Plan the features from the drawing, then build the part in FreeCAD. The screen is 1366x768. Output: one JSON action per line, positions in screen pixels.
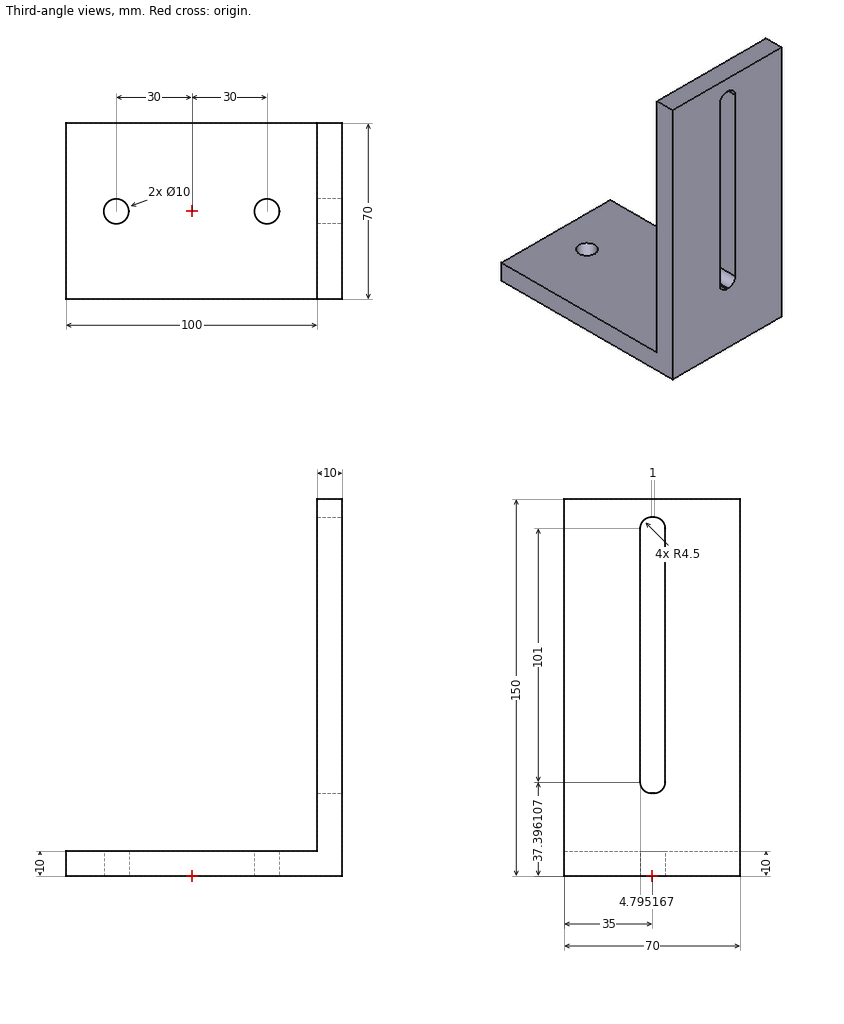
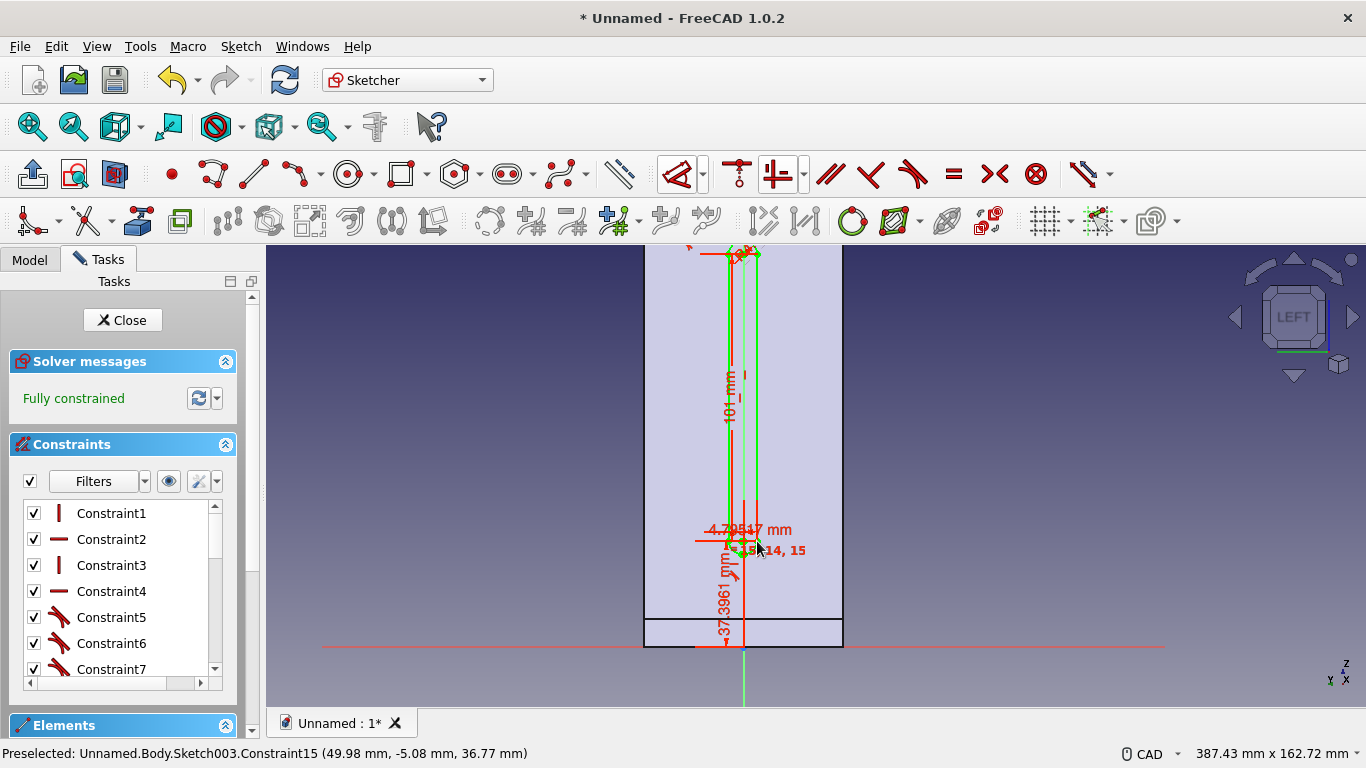
{"action": "left_click", "coordinate": [123, 320]}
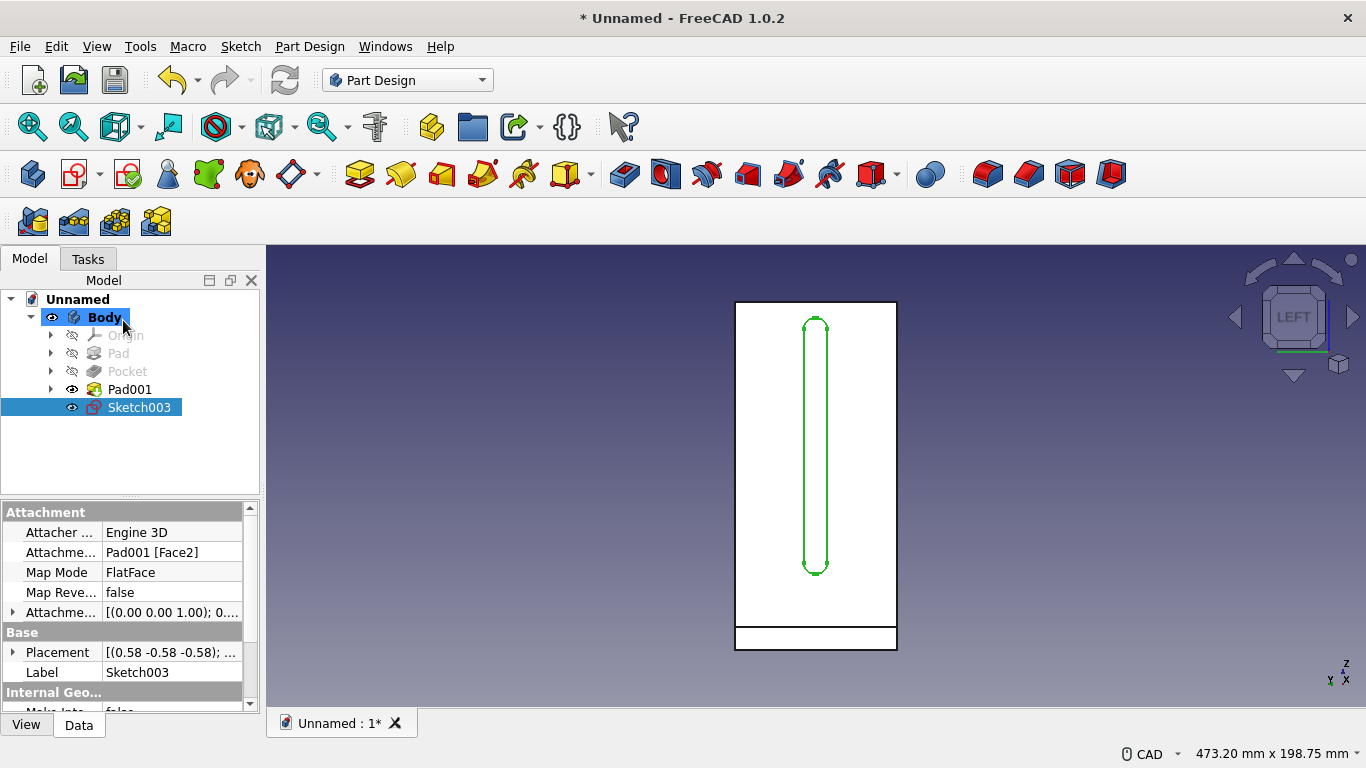
{"action": "left_click", "coordinate": [625, 174]}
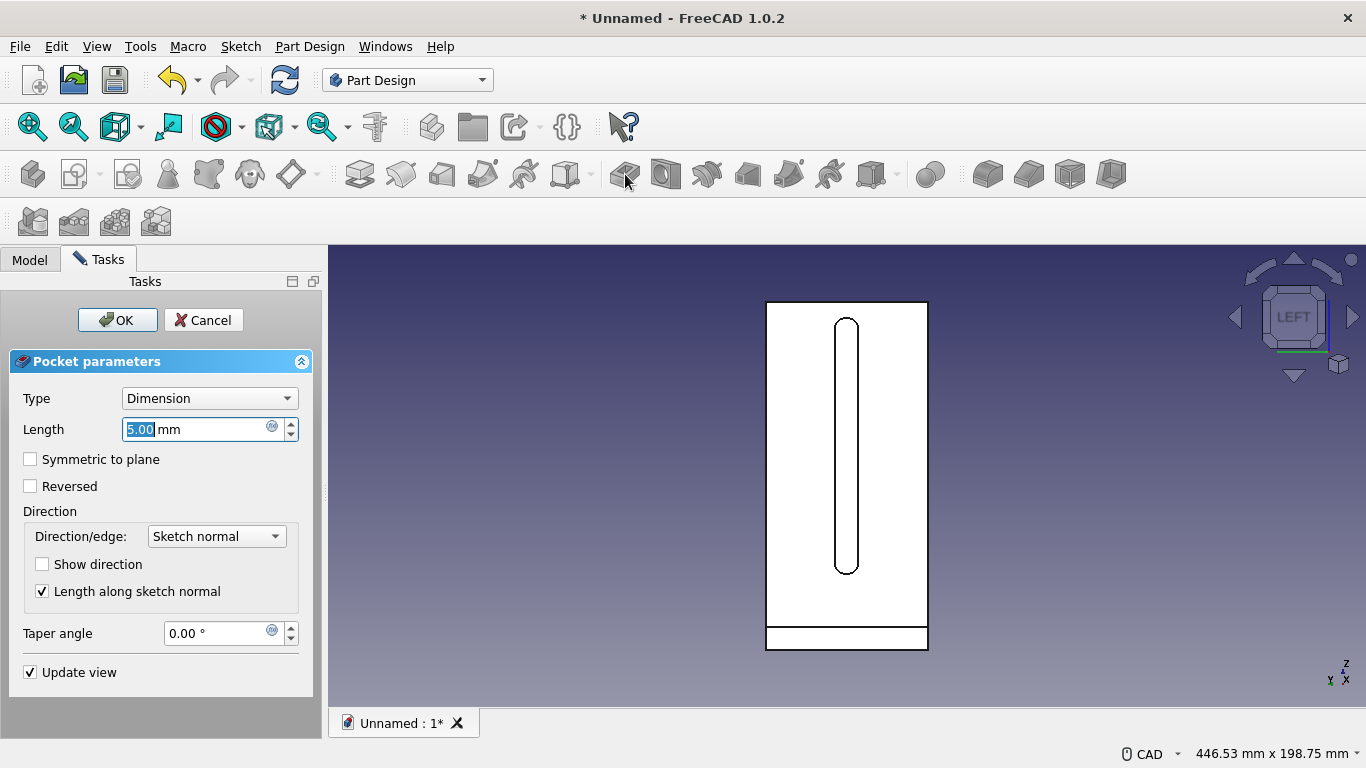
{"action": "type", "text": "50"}
{"action": "key", "text": "Tab"}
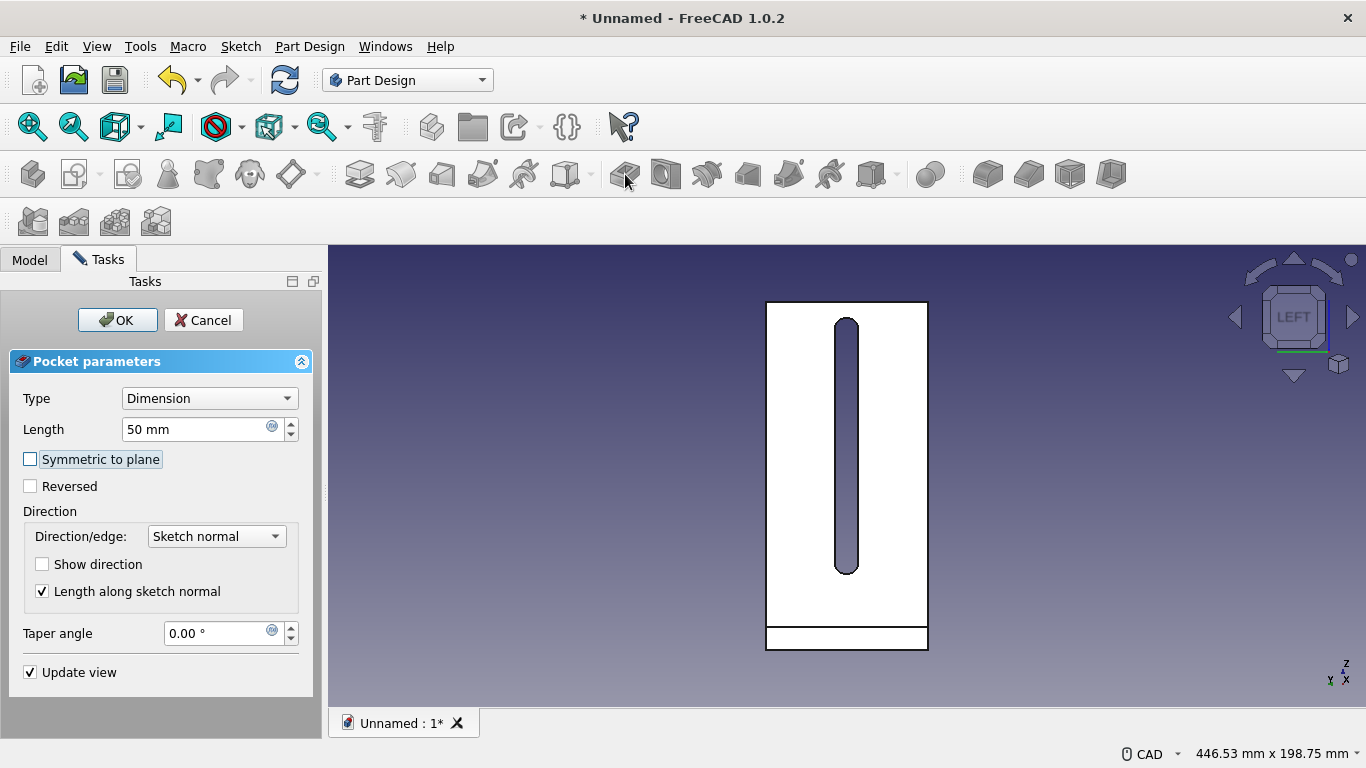
{"action": "left_click", "coordinate": [118, 320]}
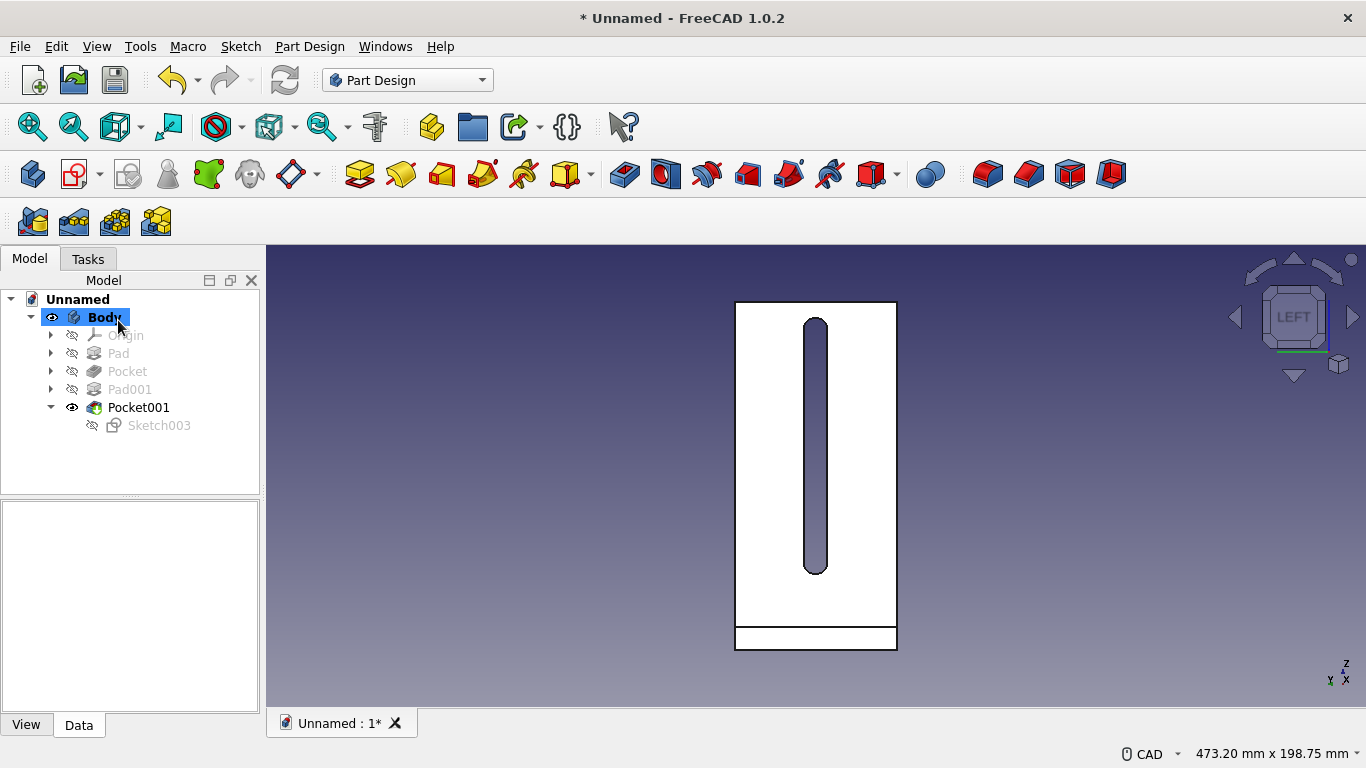
{"action": "key", "text": "0"}